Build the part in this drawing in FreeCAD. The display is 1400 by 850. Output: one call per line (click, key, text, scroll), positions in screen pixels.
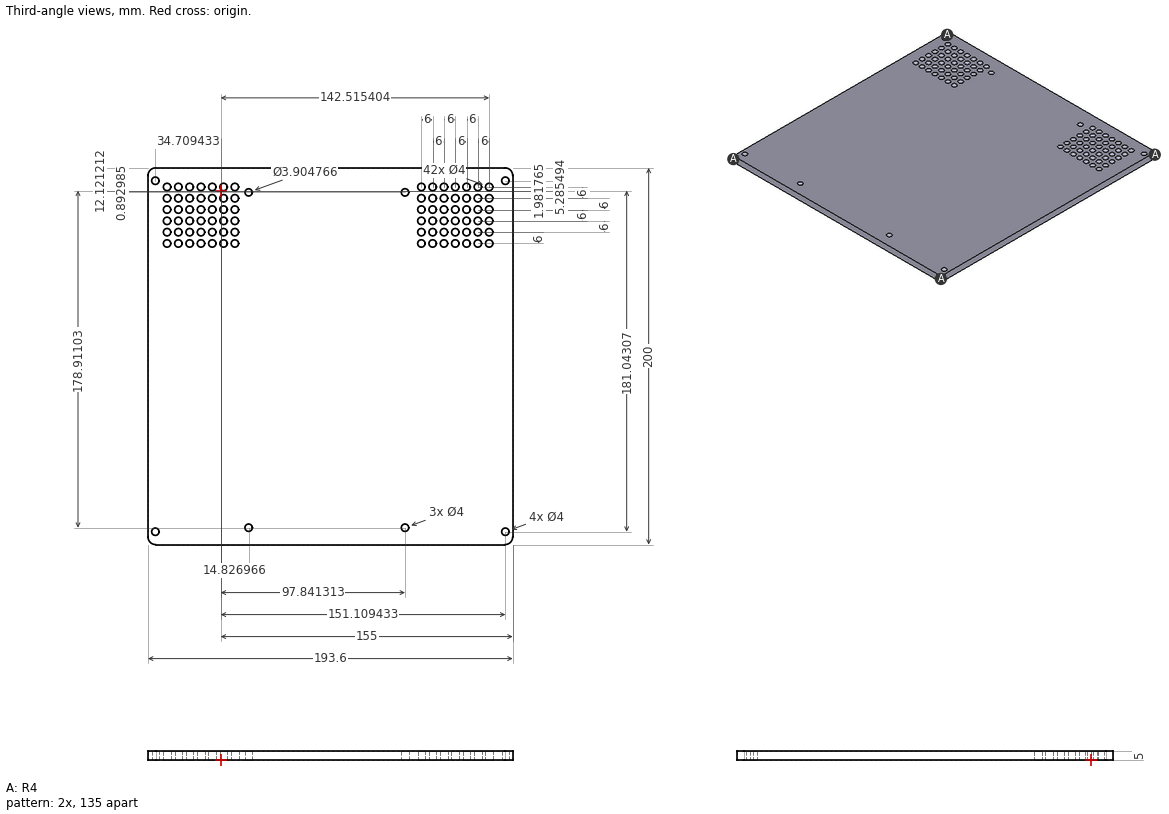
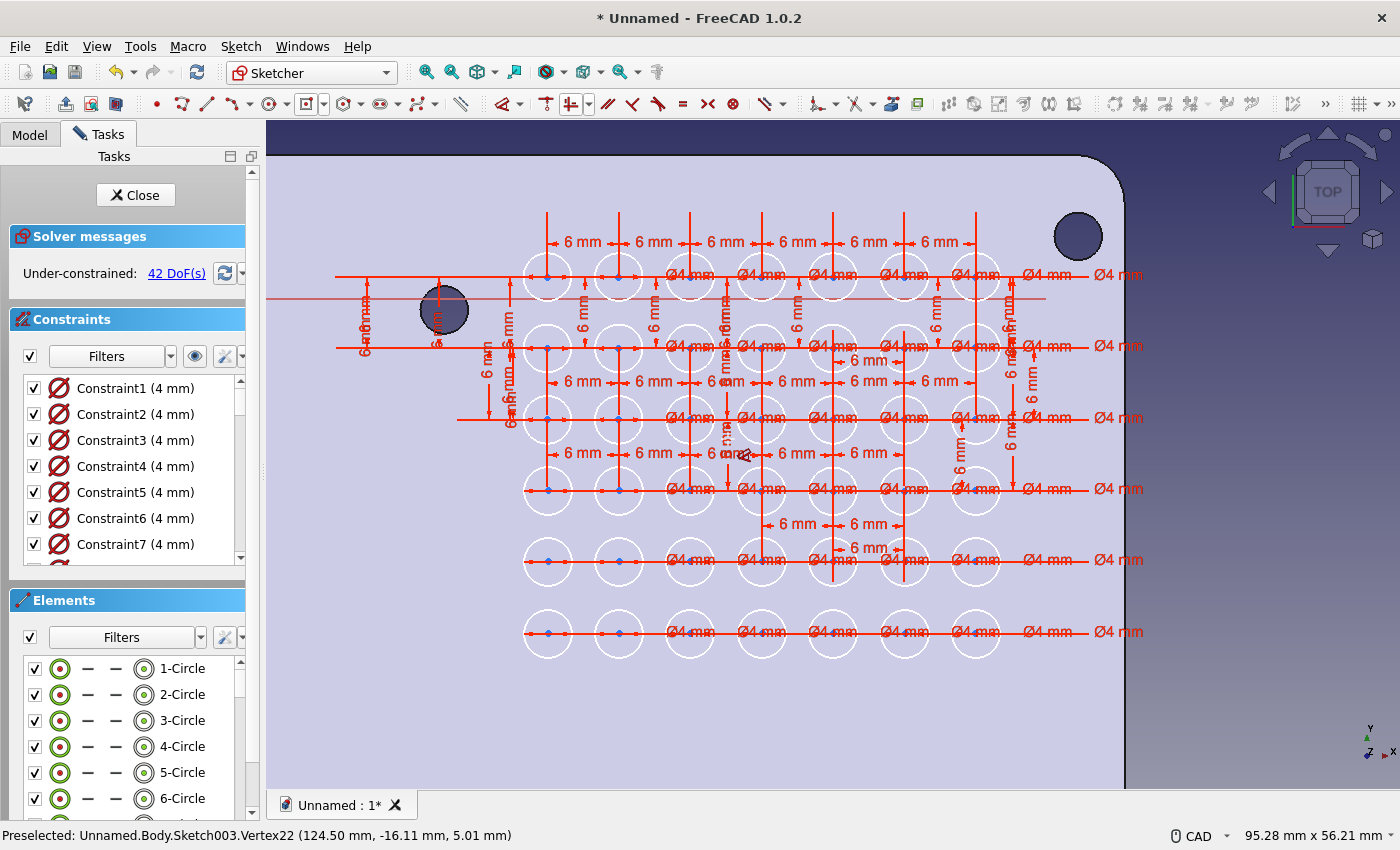
click(762, 491)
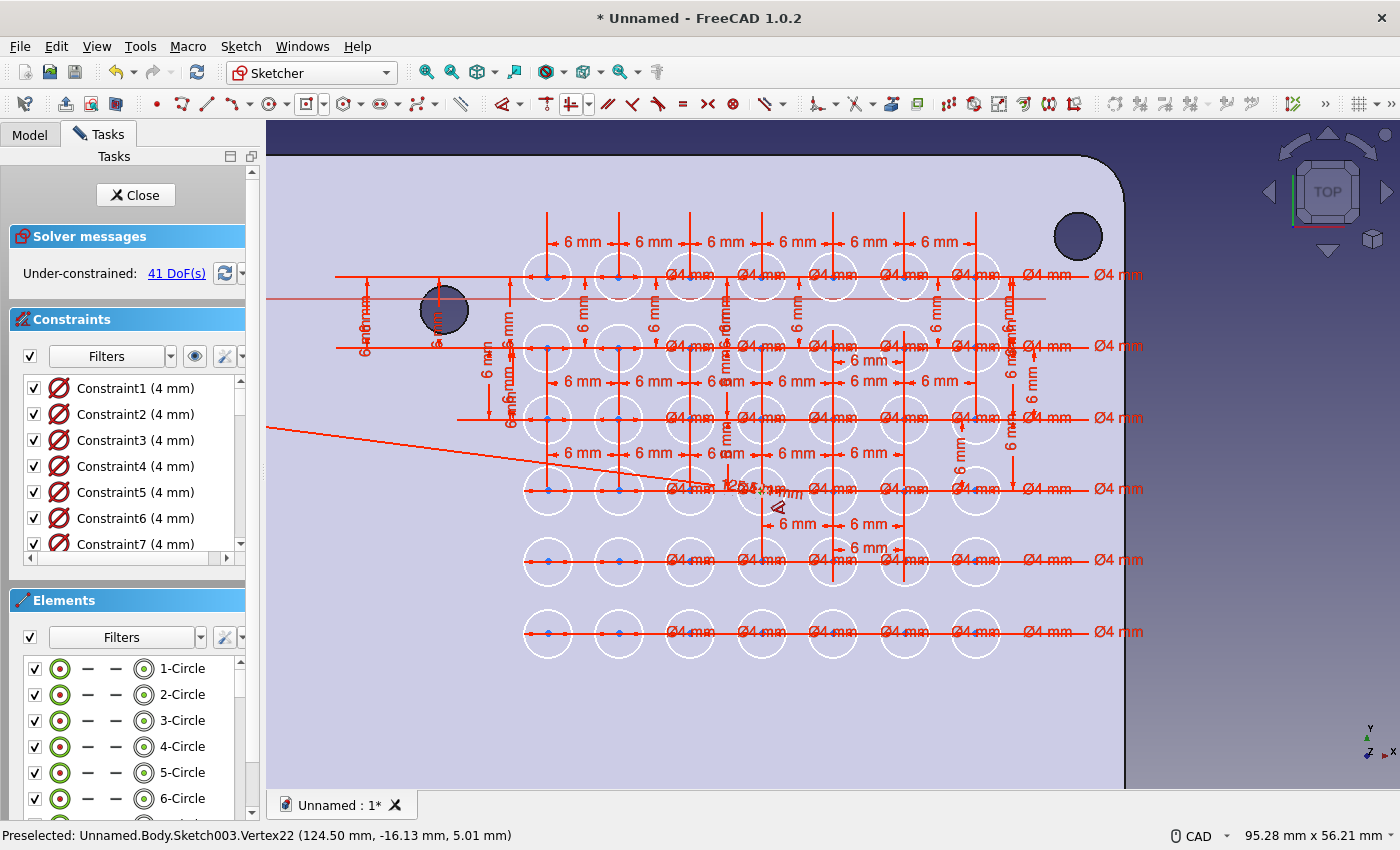
click(690, 491)
click(726, 525)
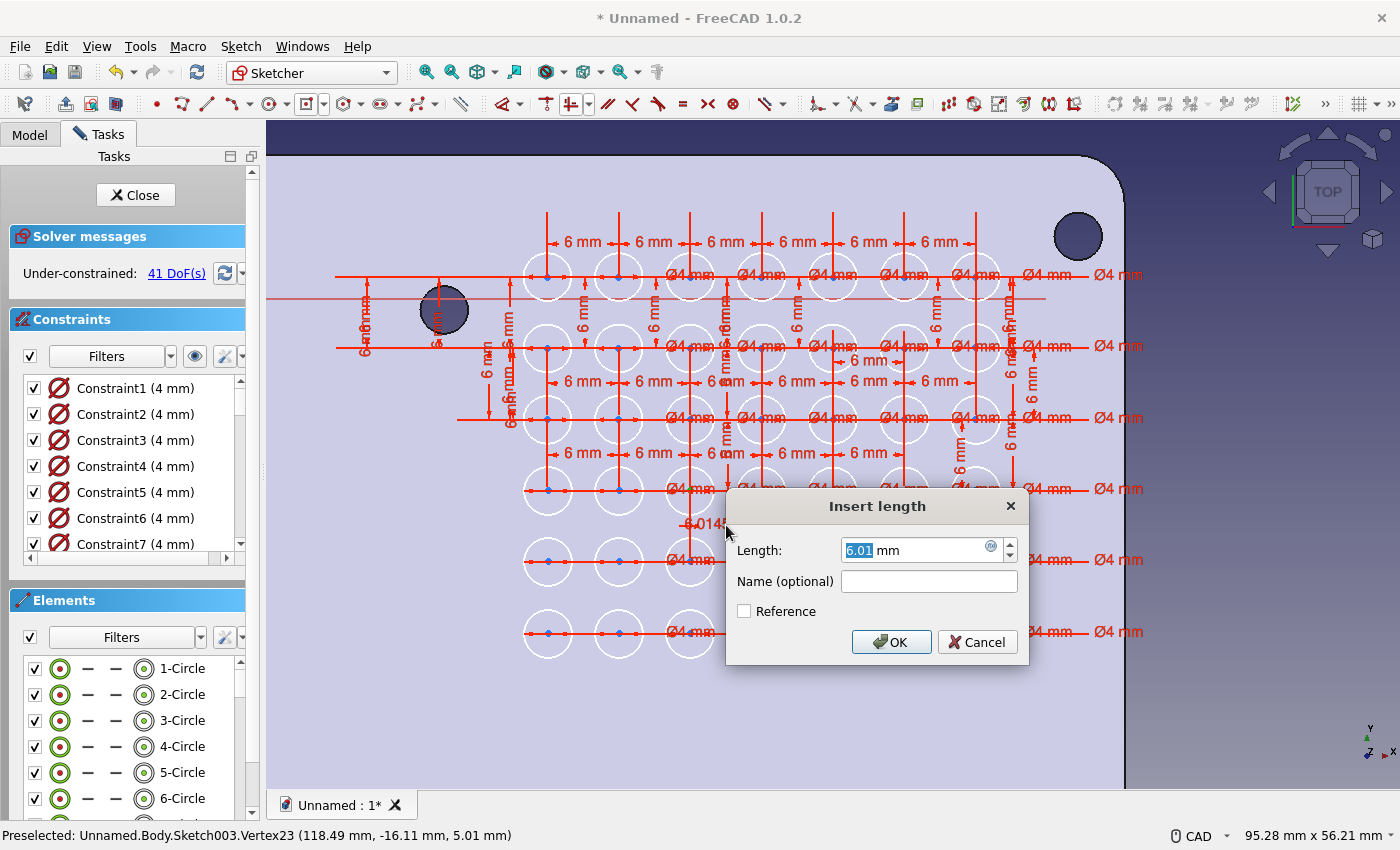
text(6)
key(Return)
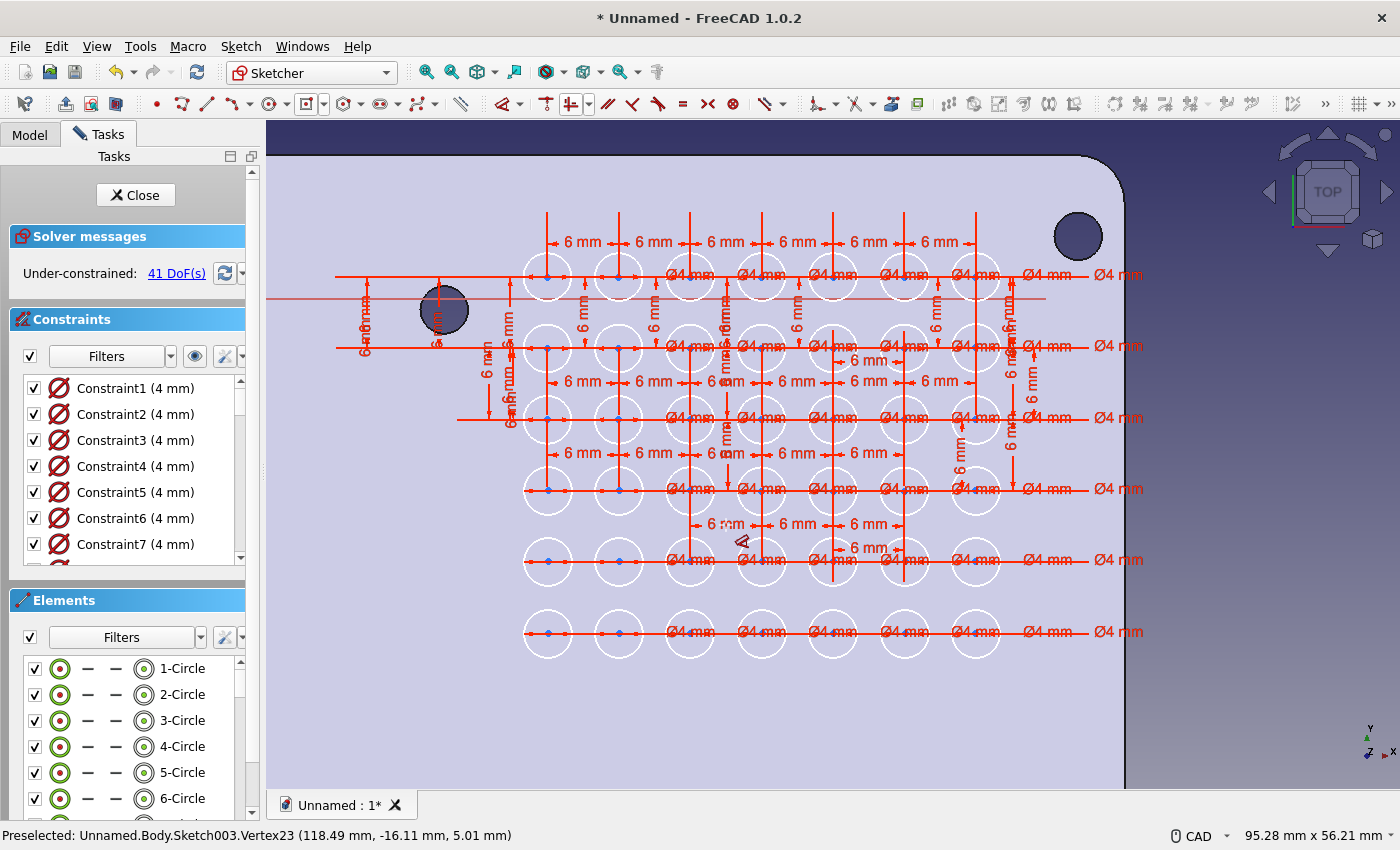
click(690, 420)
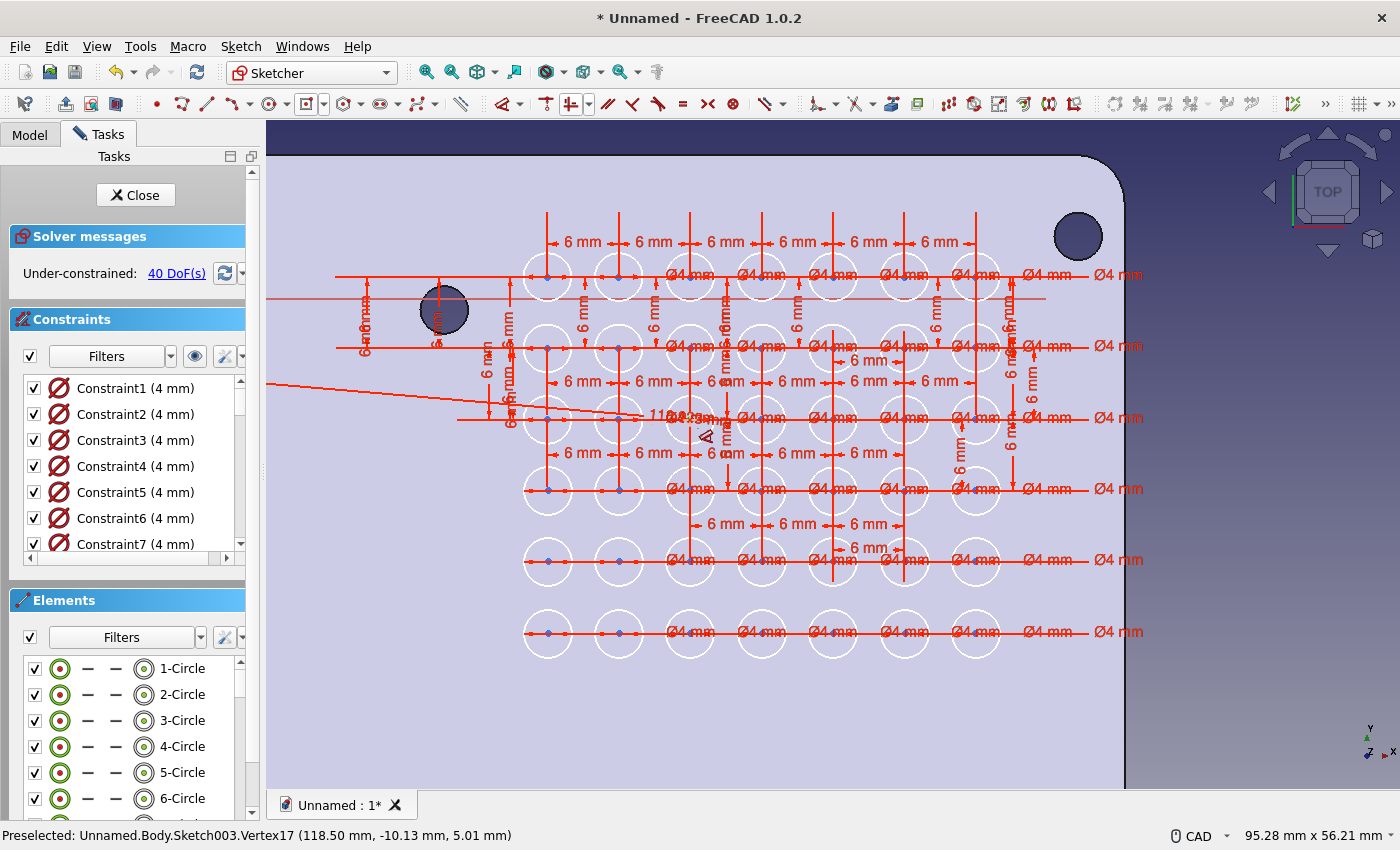
click(690, 491)
click(510, 455)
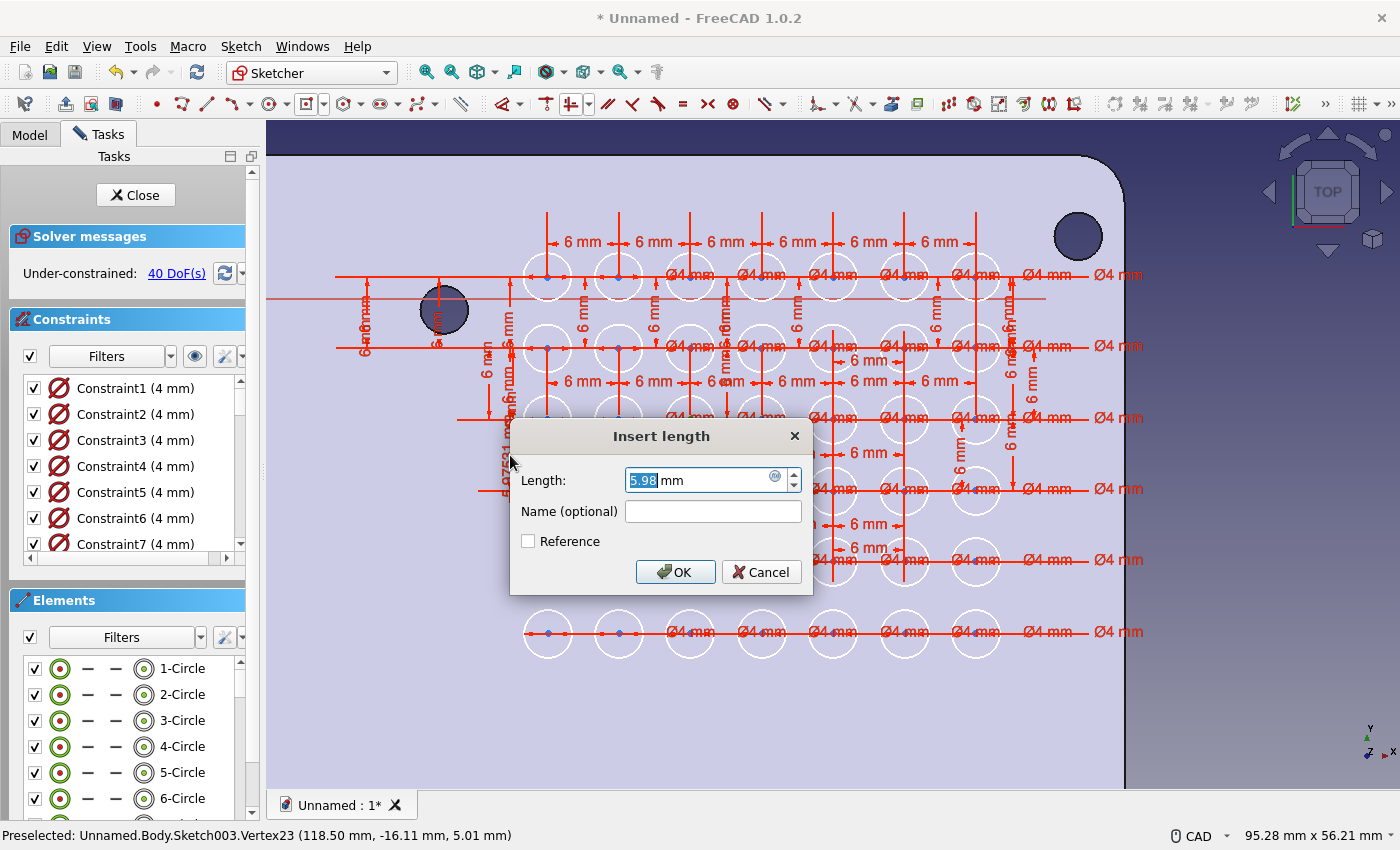
text(6)
key(Return)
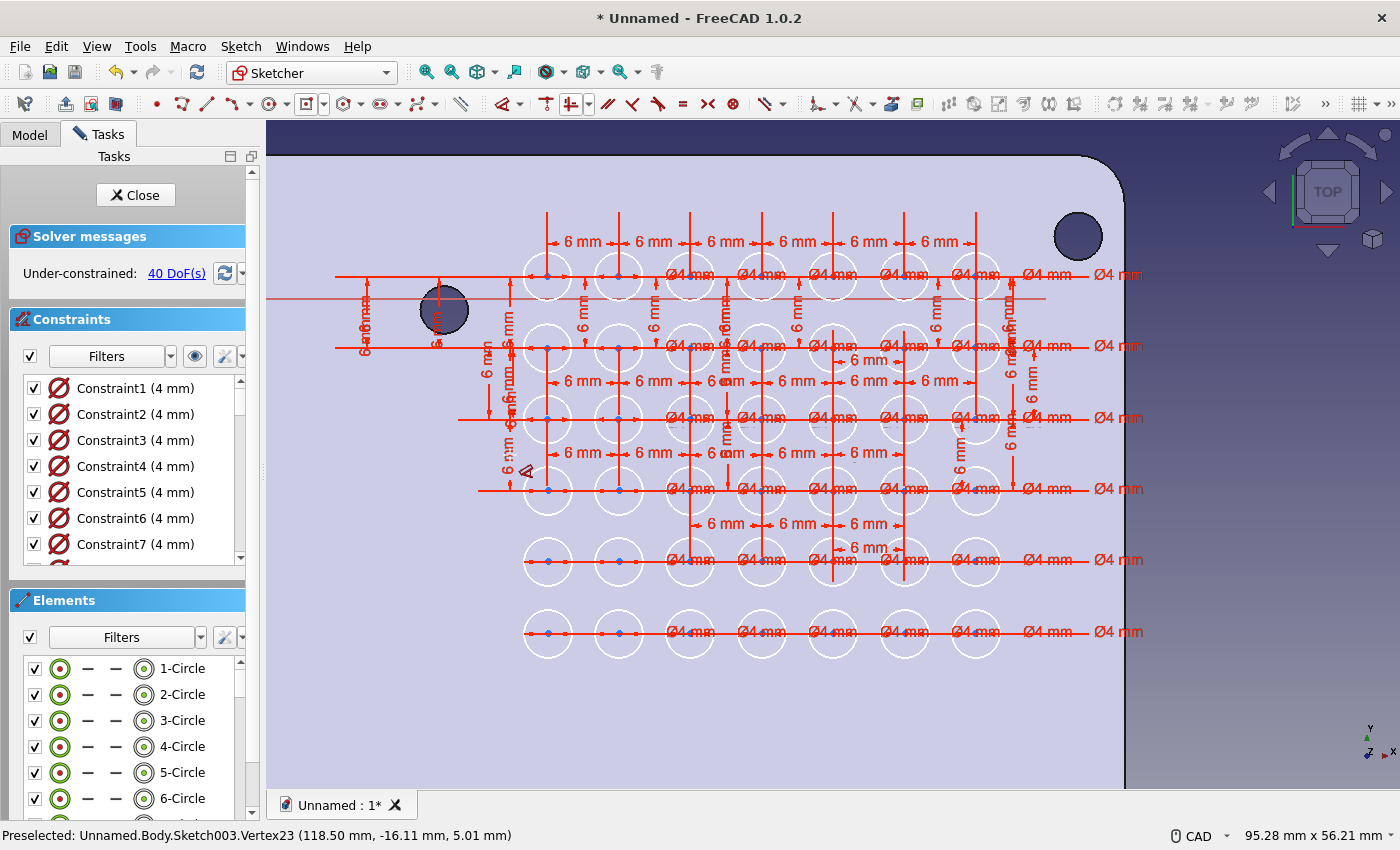
click(690, 491)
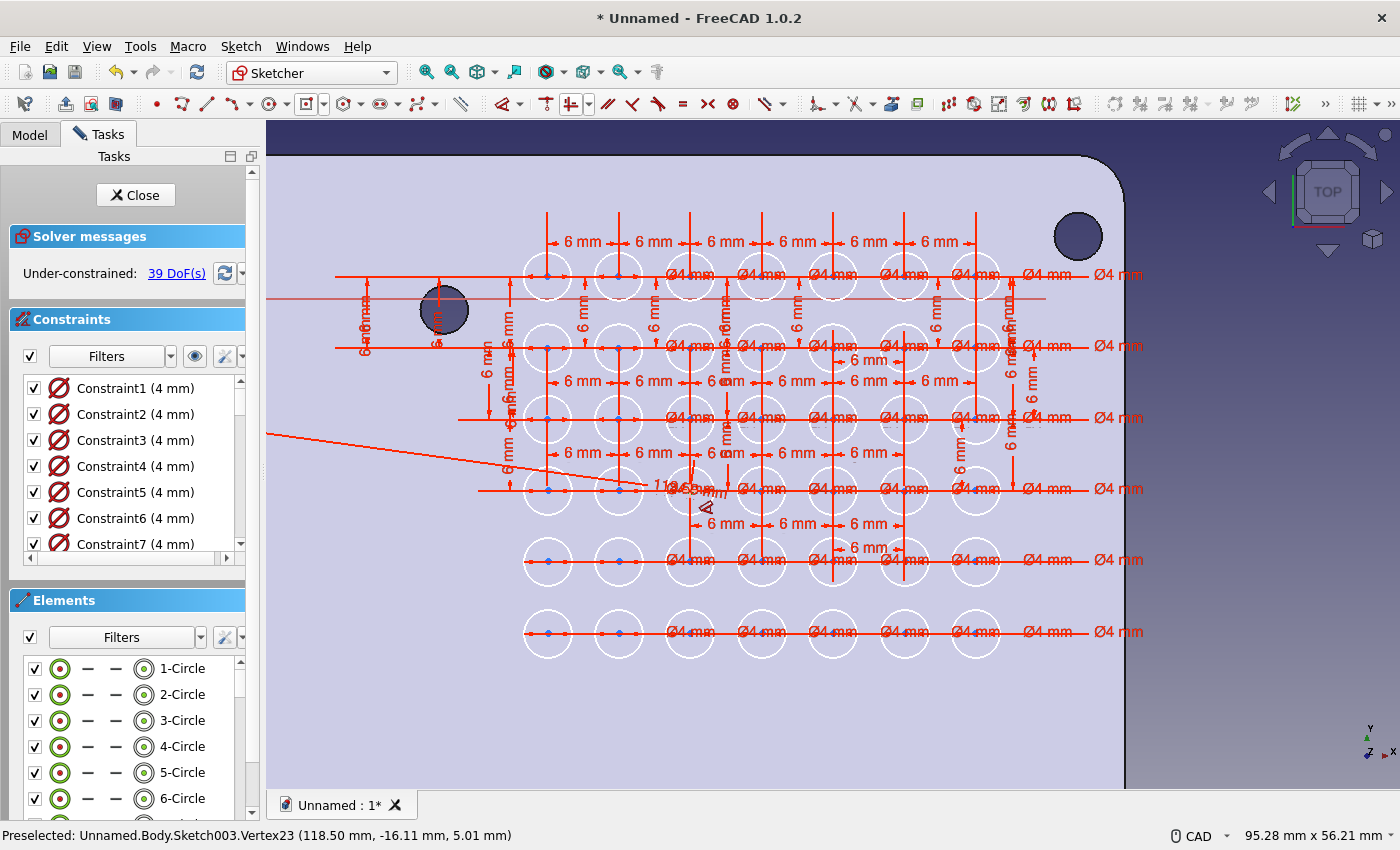
click(619, 491)
click(655, 525)